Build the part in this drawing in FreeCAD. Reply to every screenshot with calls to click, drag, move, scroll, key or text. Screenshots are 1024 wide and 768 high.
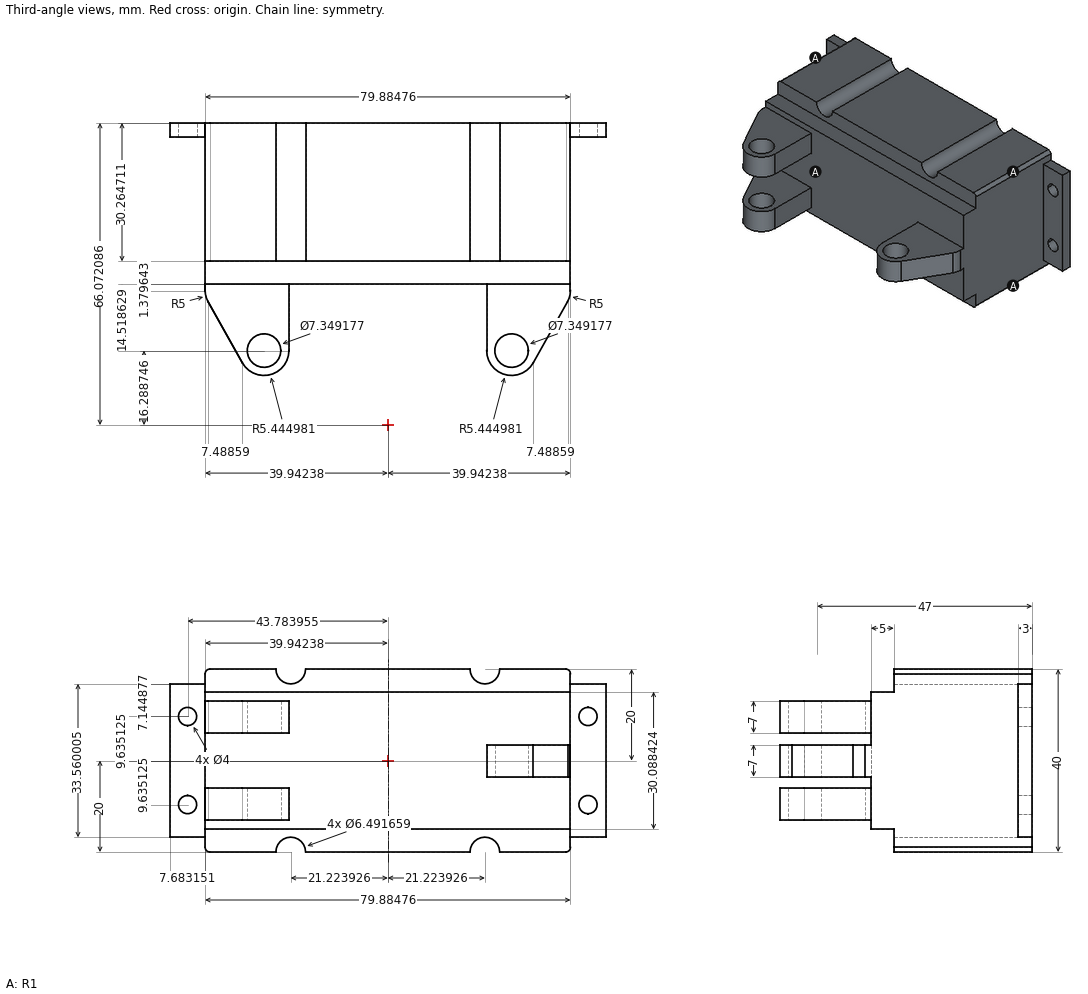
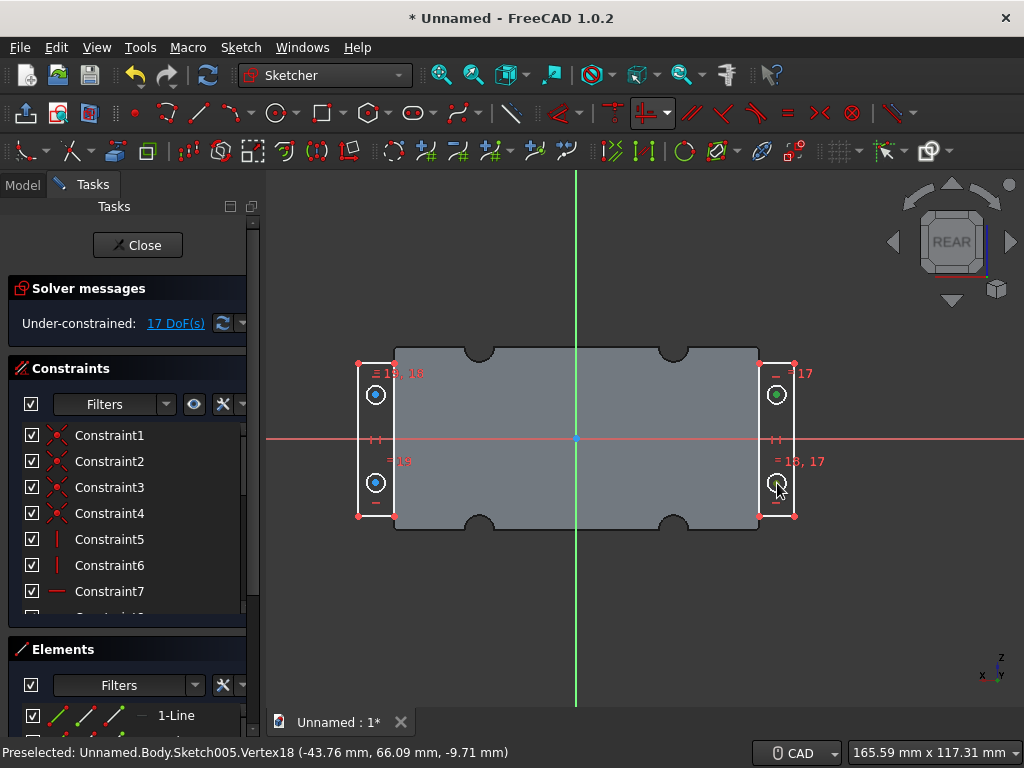
key(v)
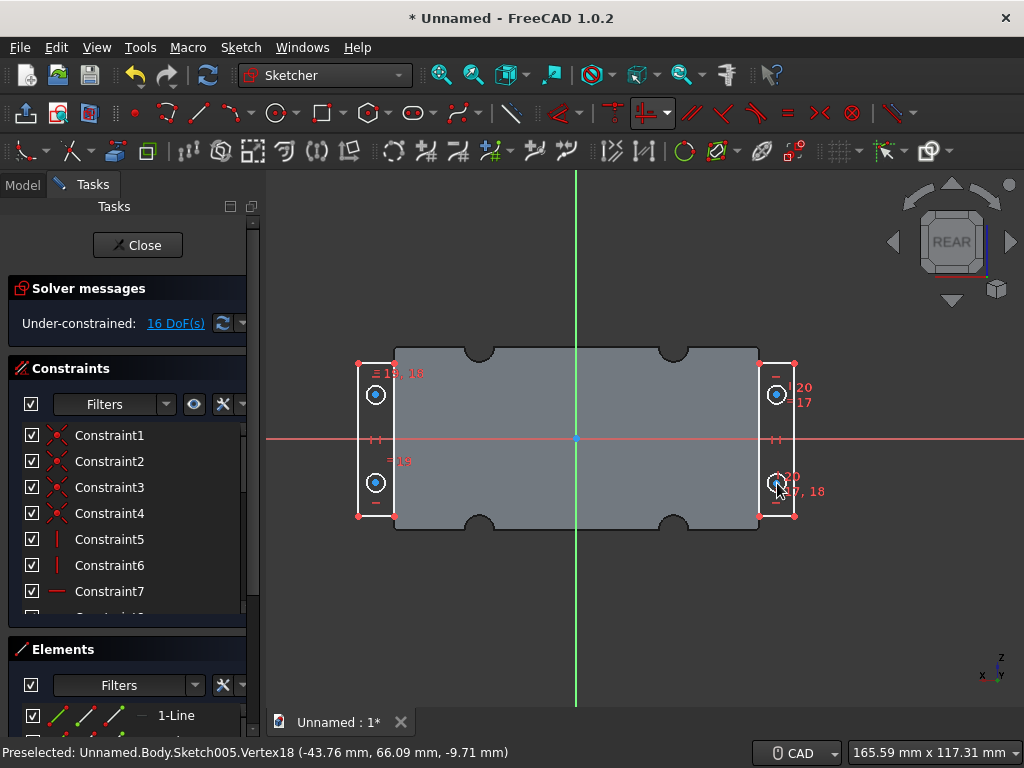
click(376, 395)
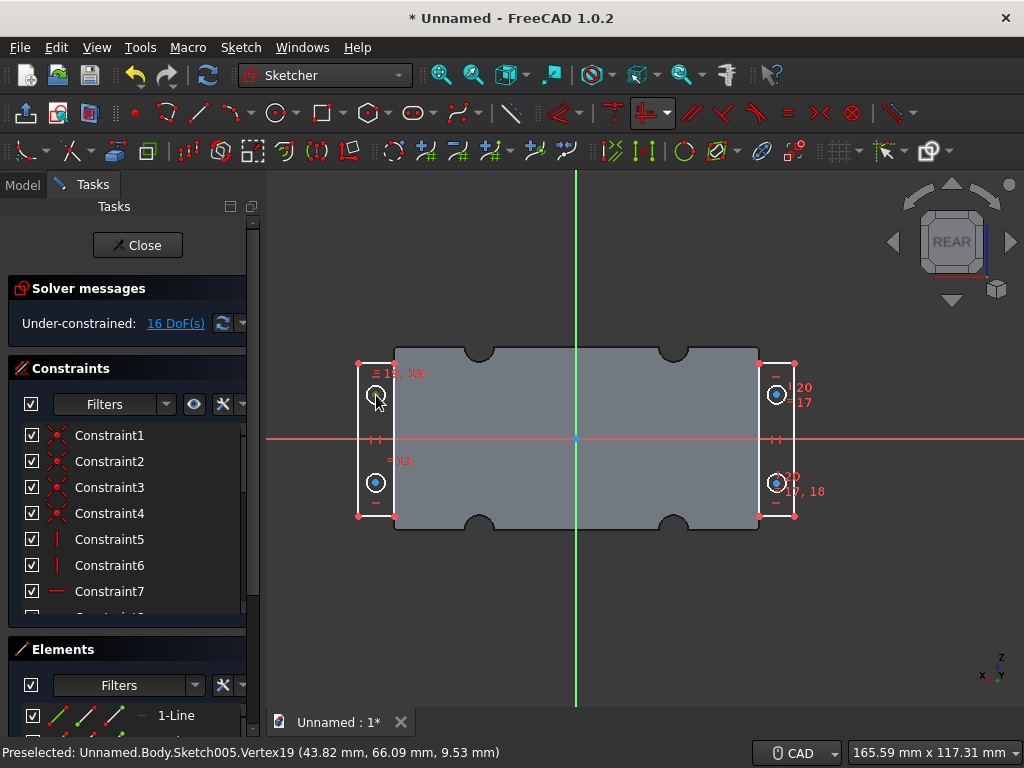
click(376, 483)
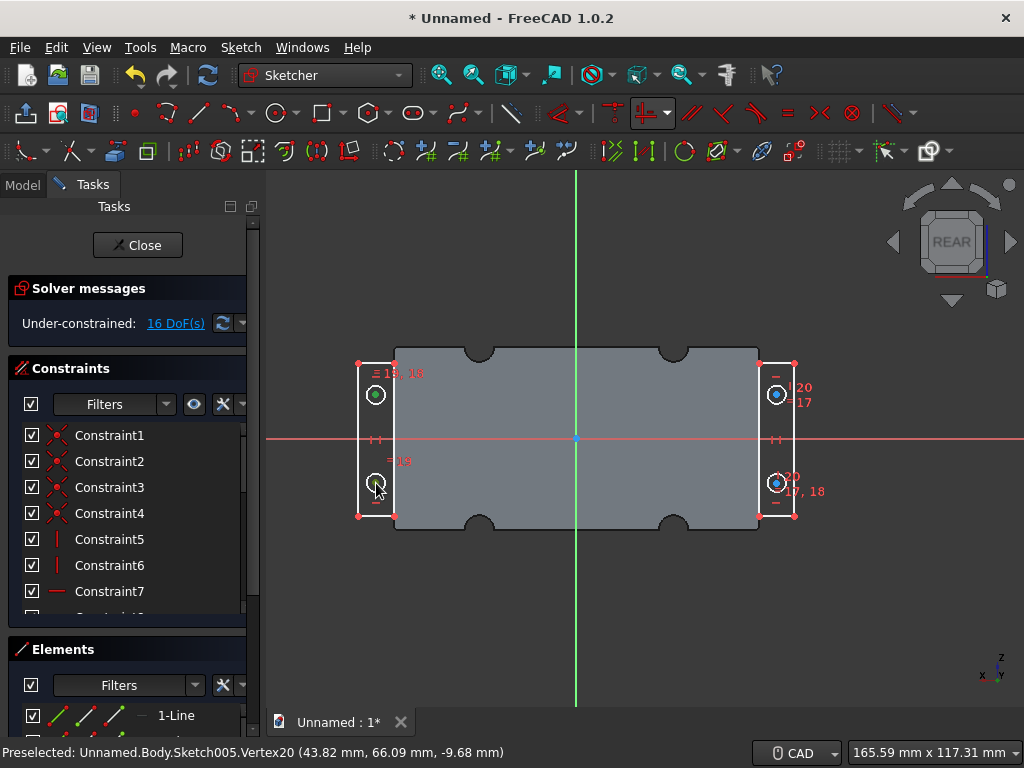
key(v)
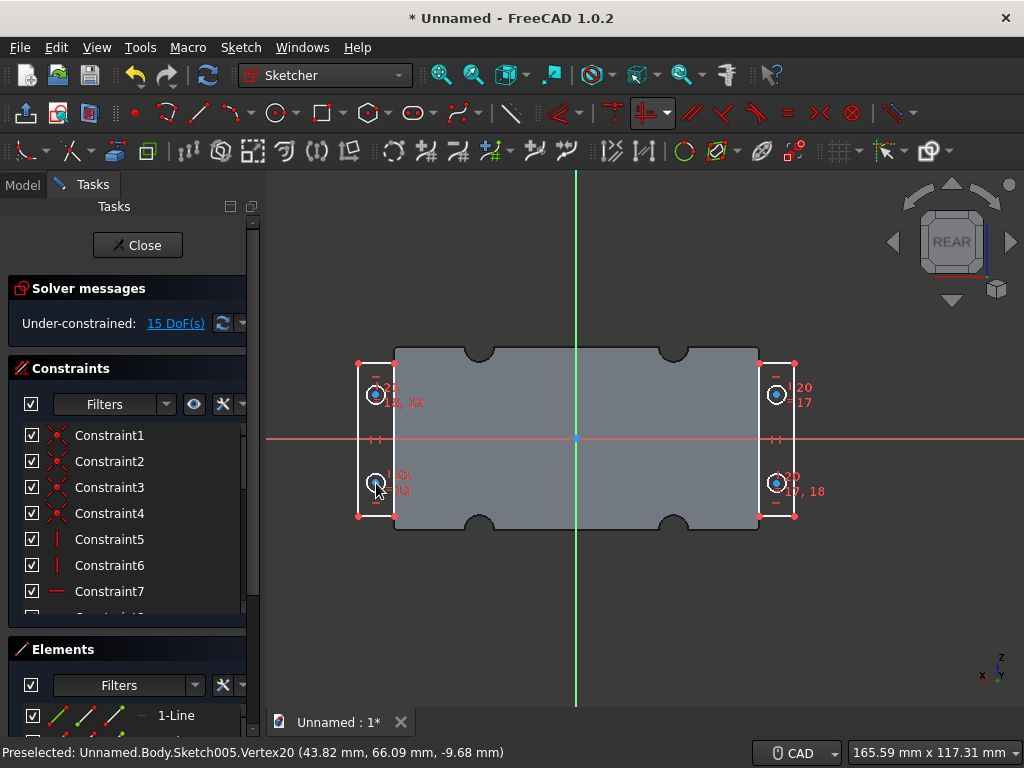
click(777, 395)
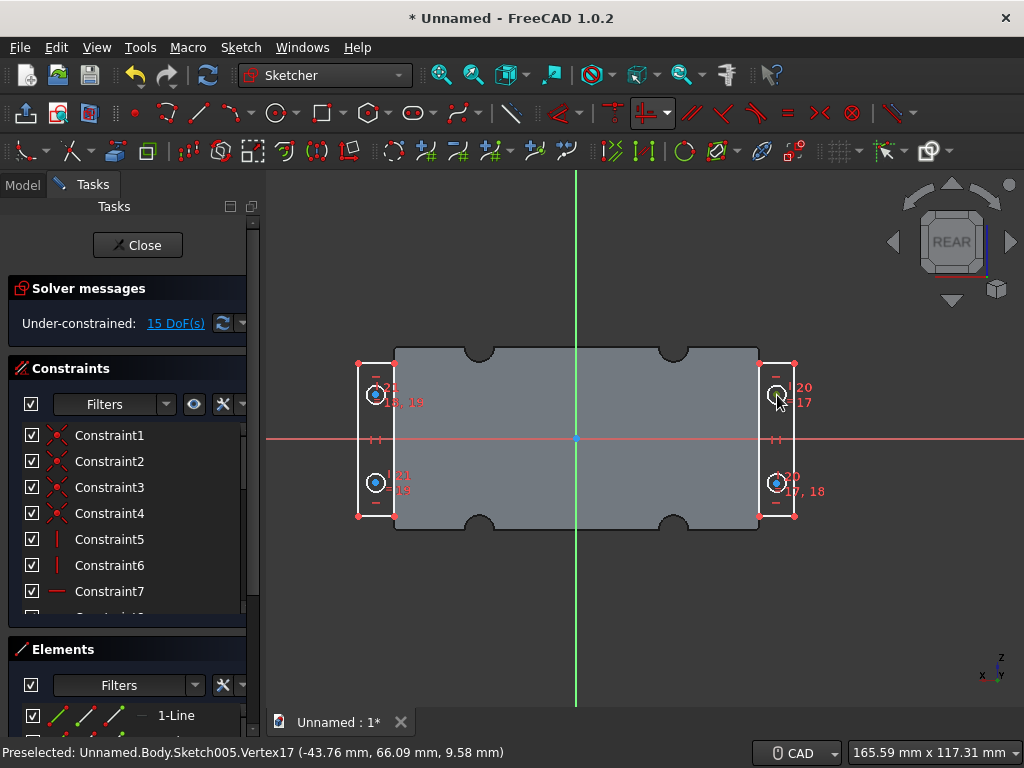
click(376, 395)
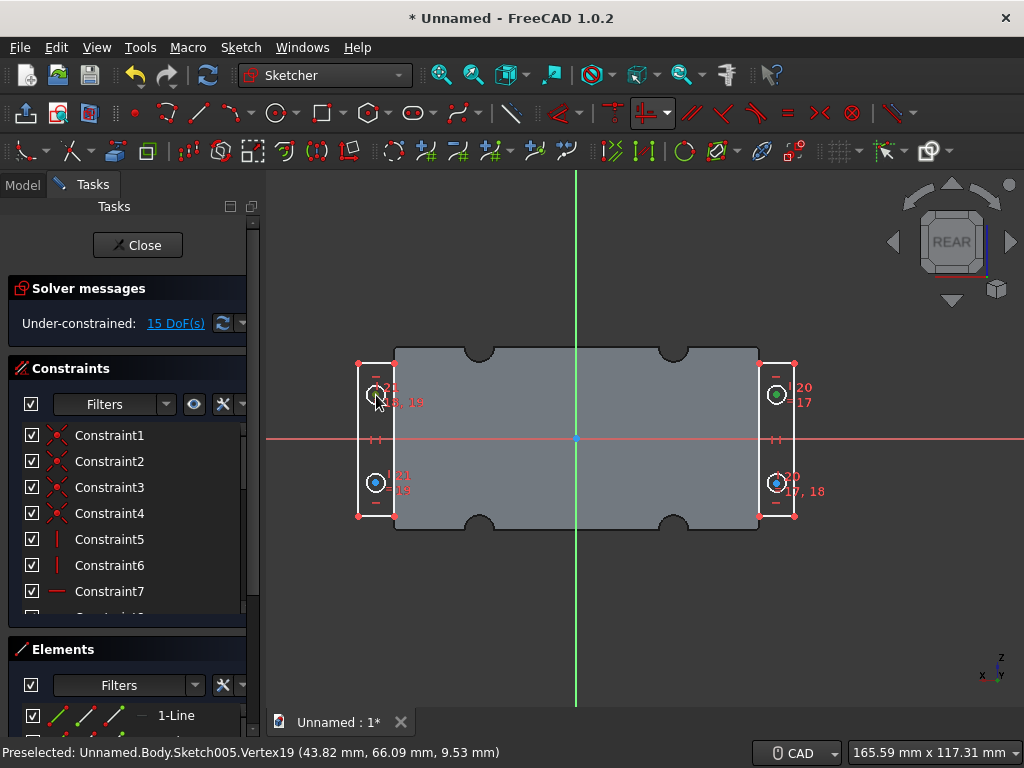
click(576, 645)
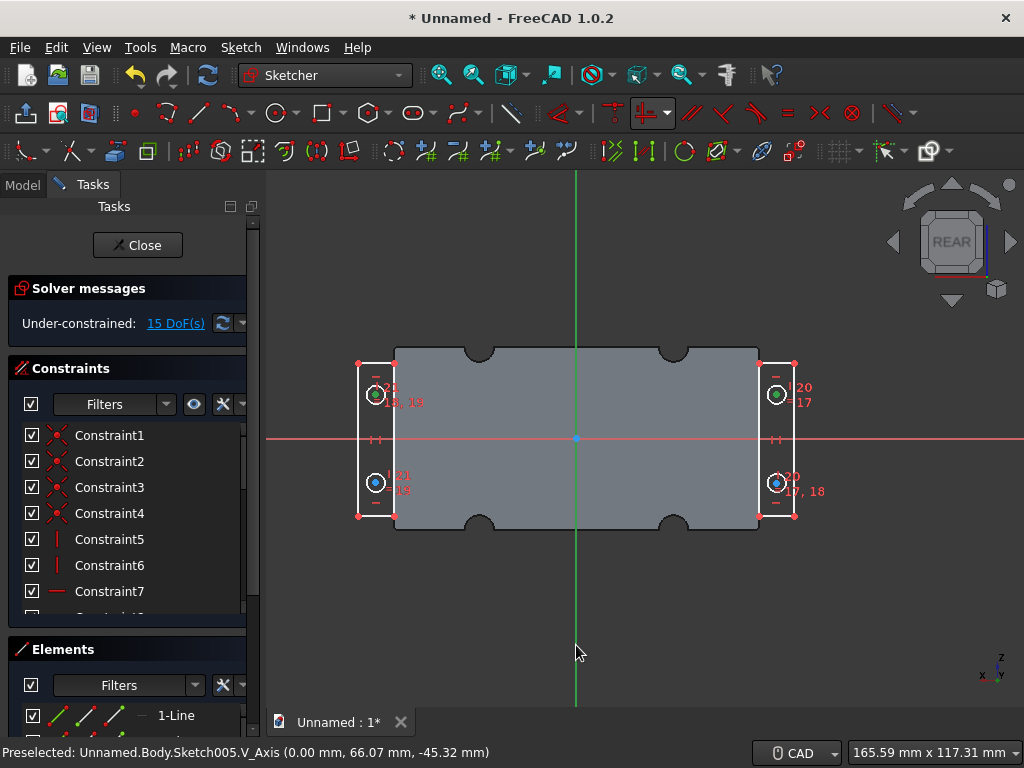
click(820, 114)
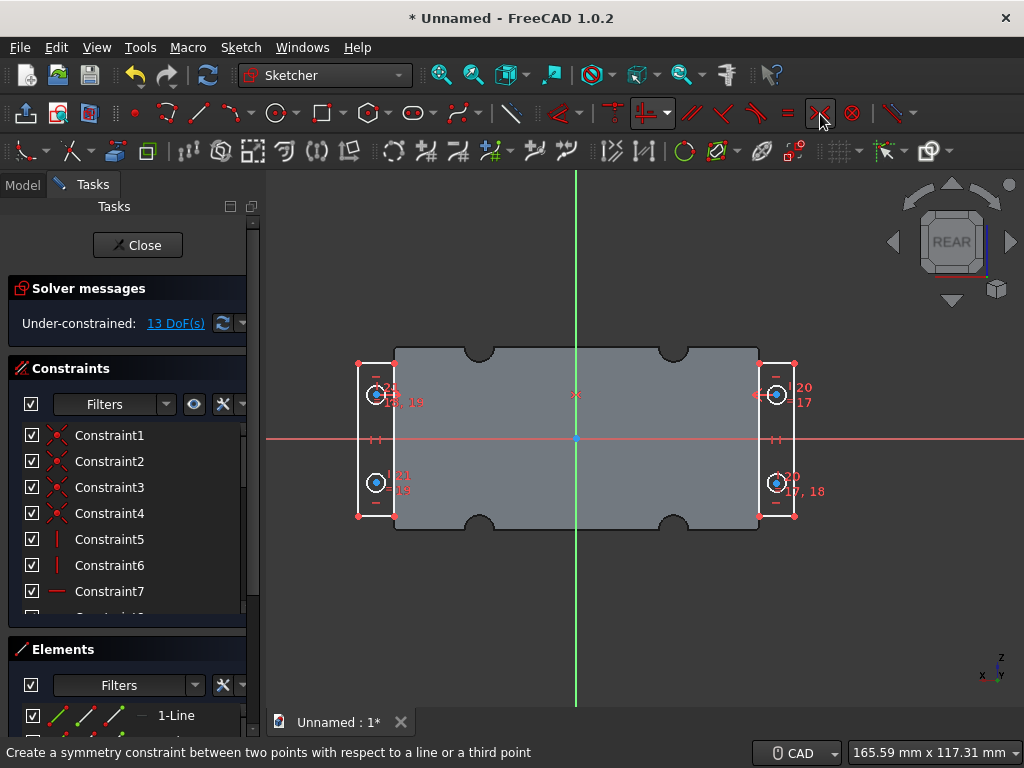
click(794, 363)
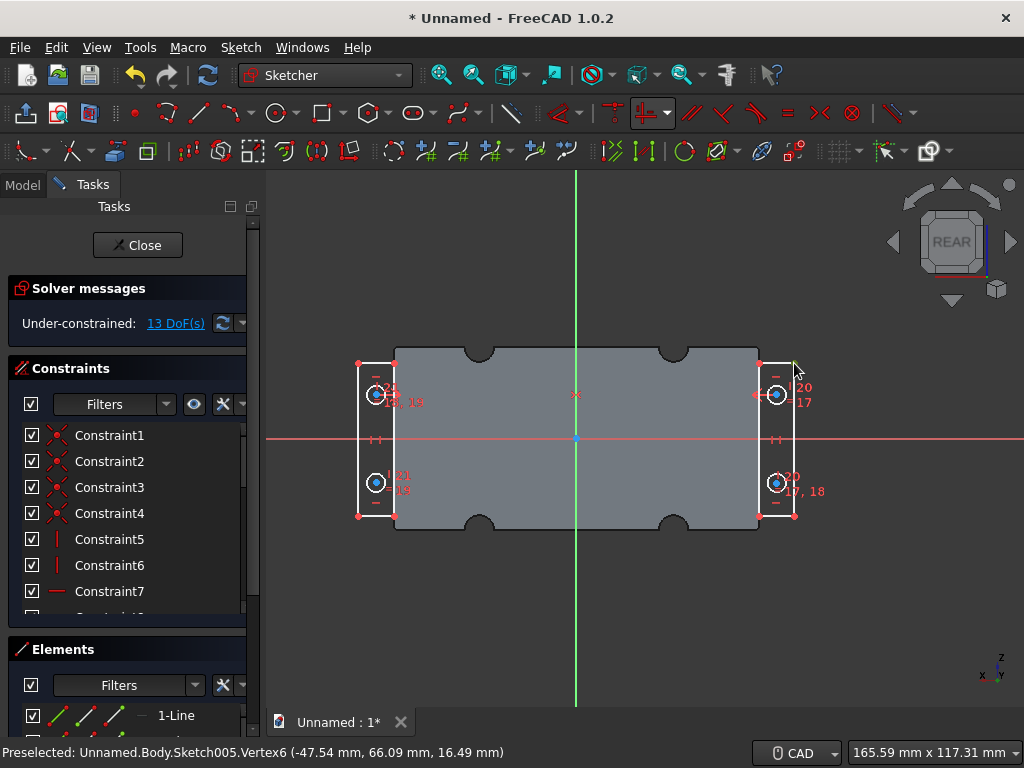
click(358, 363)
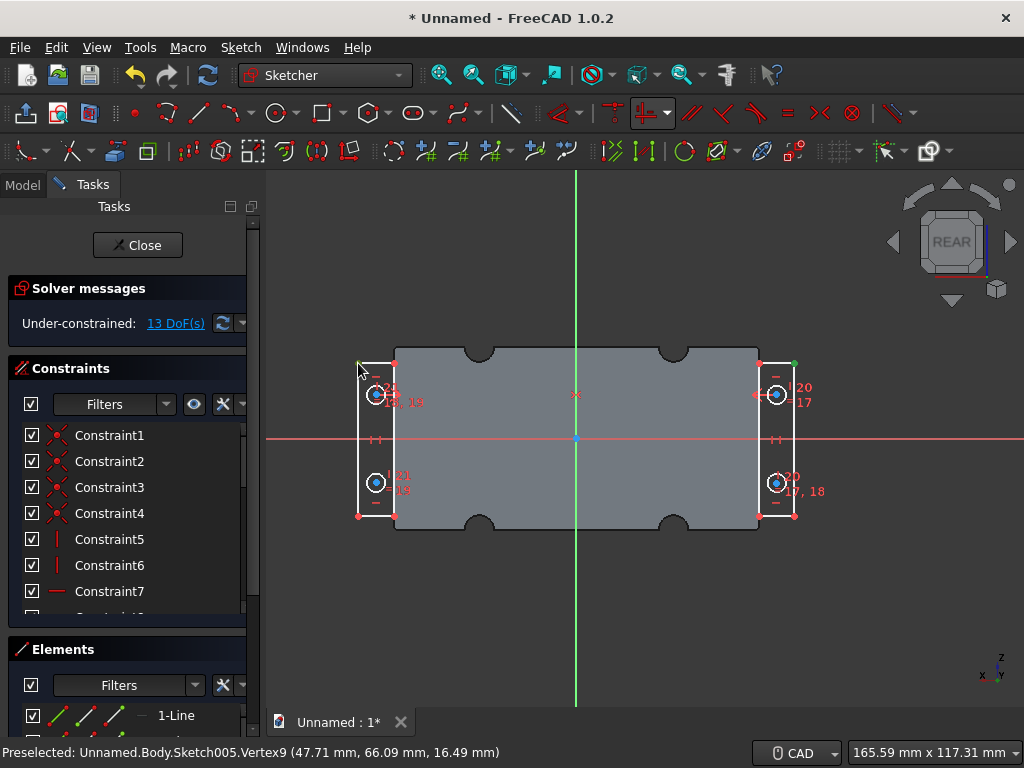
click(576, 645)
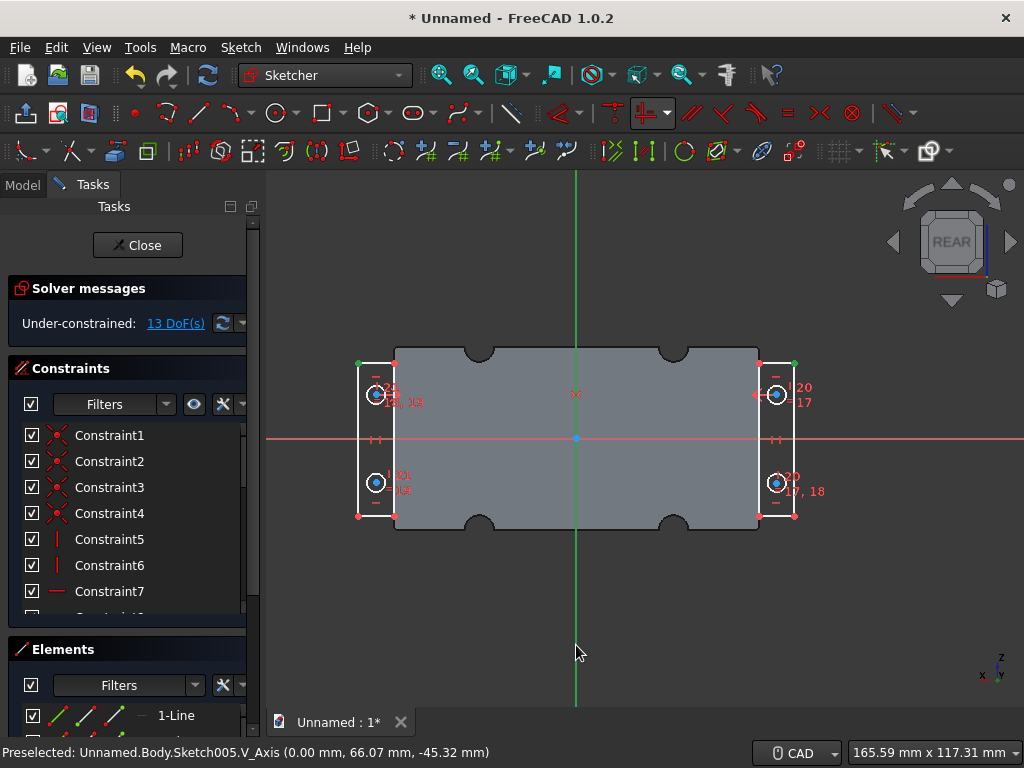
click(820, 114)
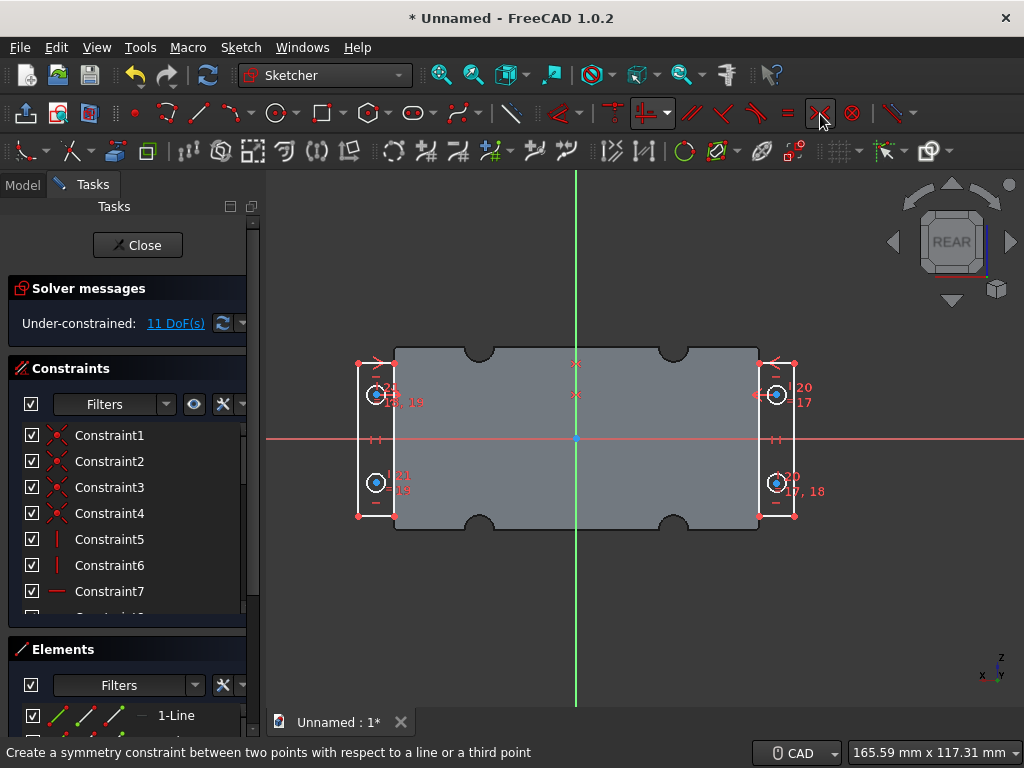
click(759, 516)